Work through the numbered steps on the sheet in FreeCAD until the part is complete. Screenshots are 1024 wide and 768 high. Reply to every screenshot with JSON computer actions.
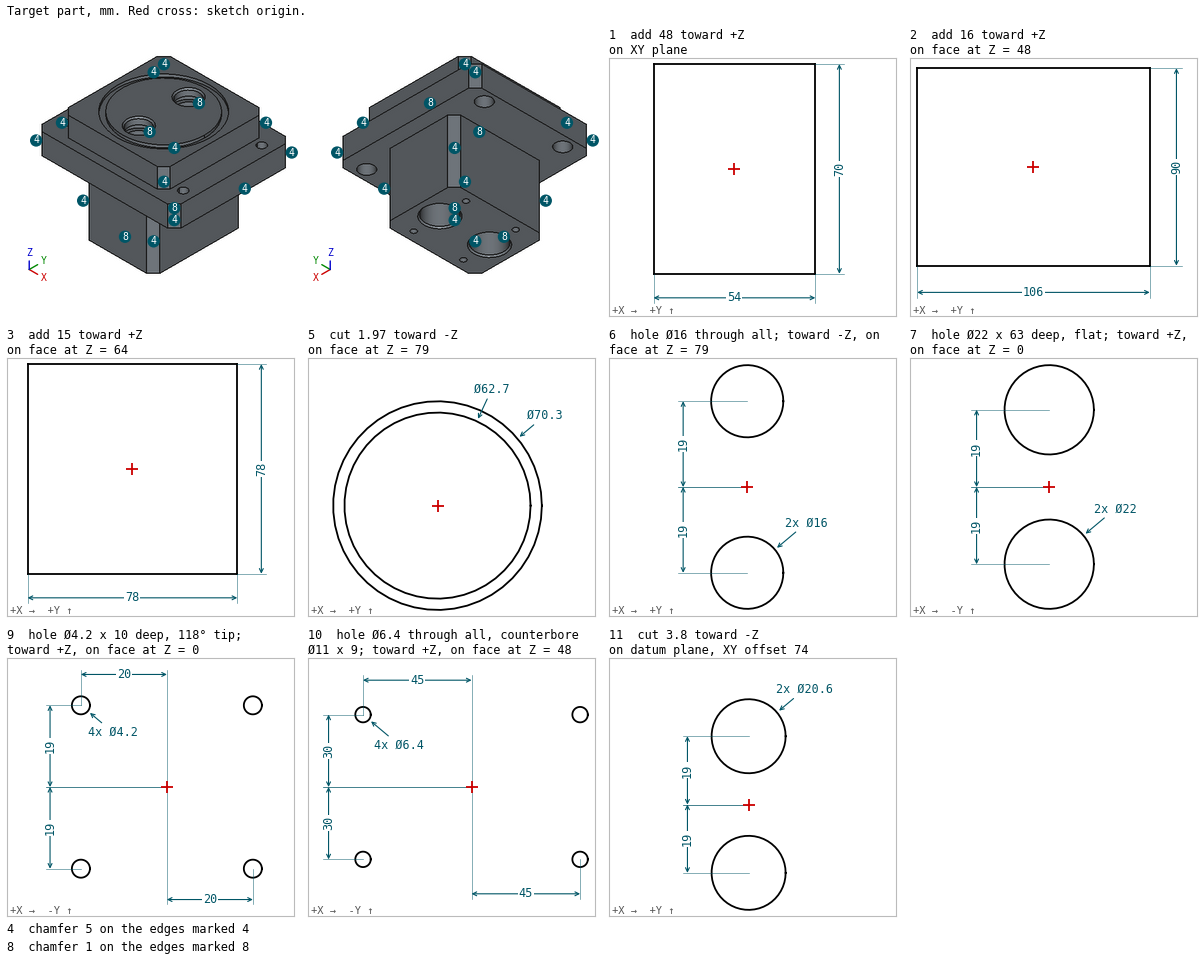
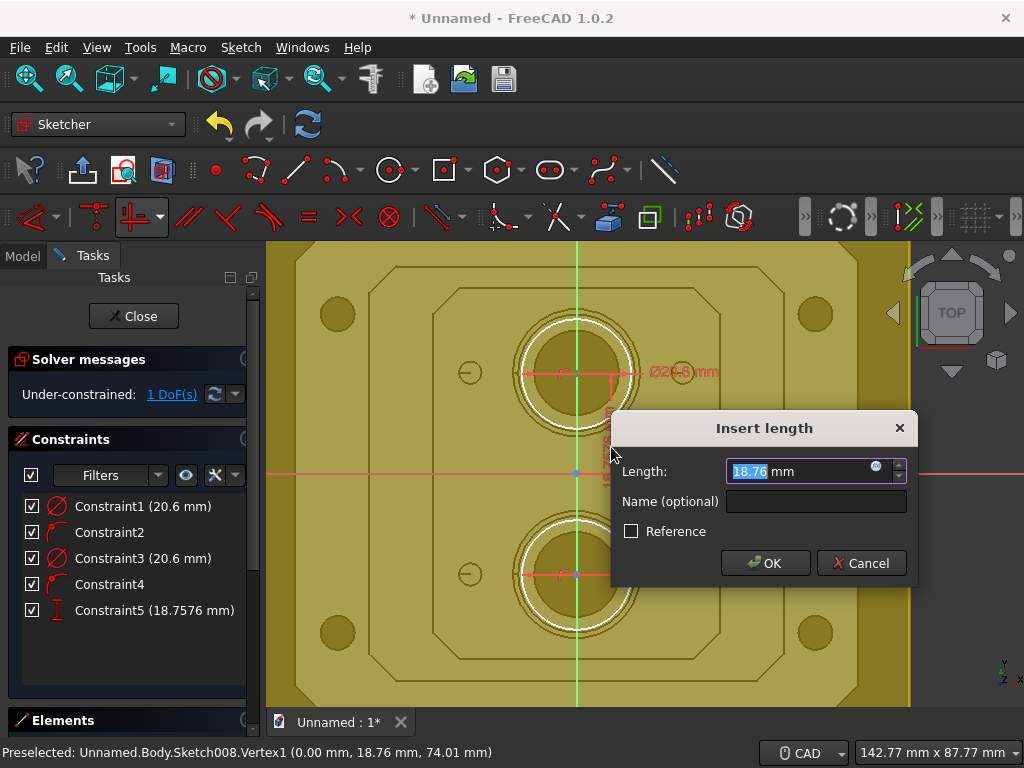
{"action": "type", "text": "19"}
{"action": "key", "text": "Return"}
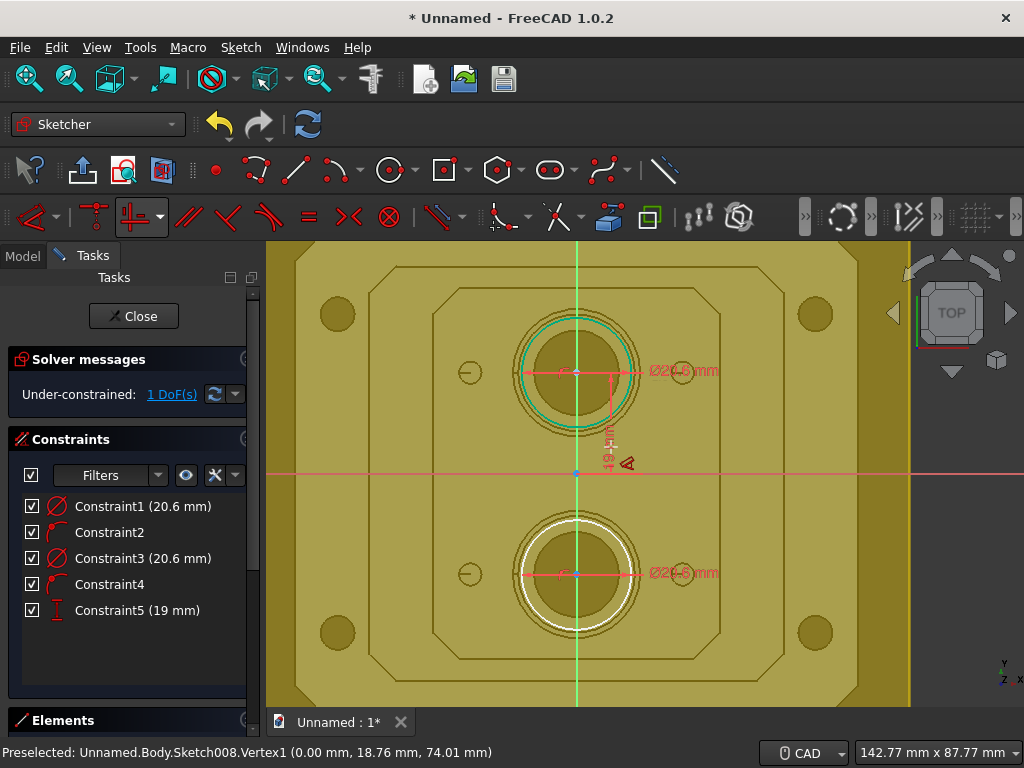
{"action": "left_click", "coordinate": [577, 575]}
{"action": "left_click", "coordinate": [611, 501]}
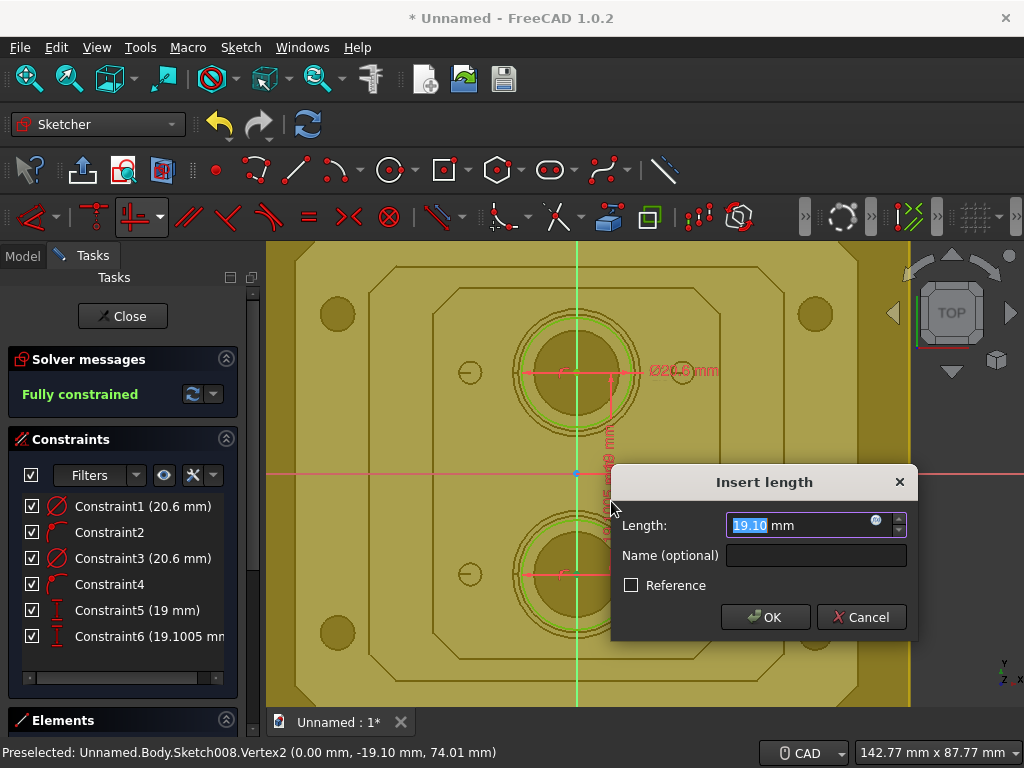
{"action": "type", "text": "19"}
{"action": "key", "text": "Return"}
{"action": "key", "text": "Escape"}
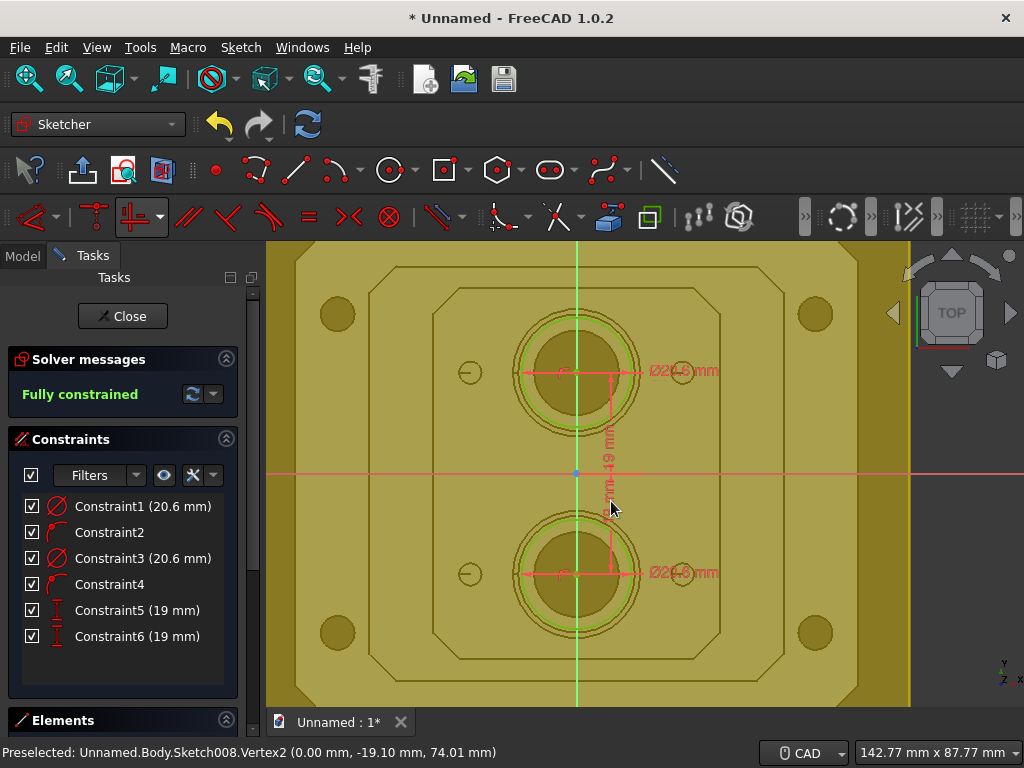
{"action": "left_click", "coordinate": [123, 316]}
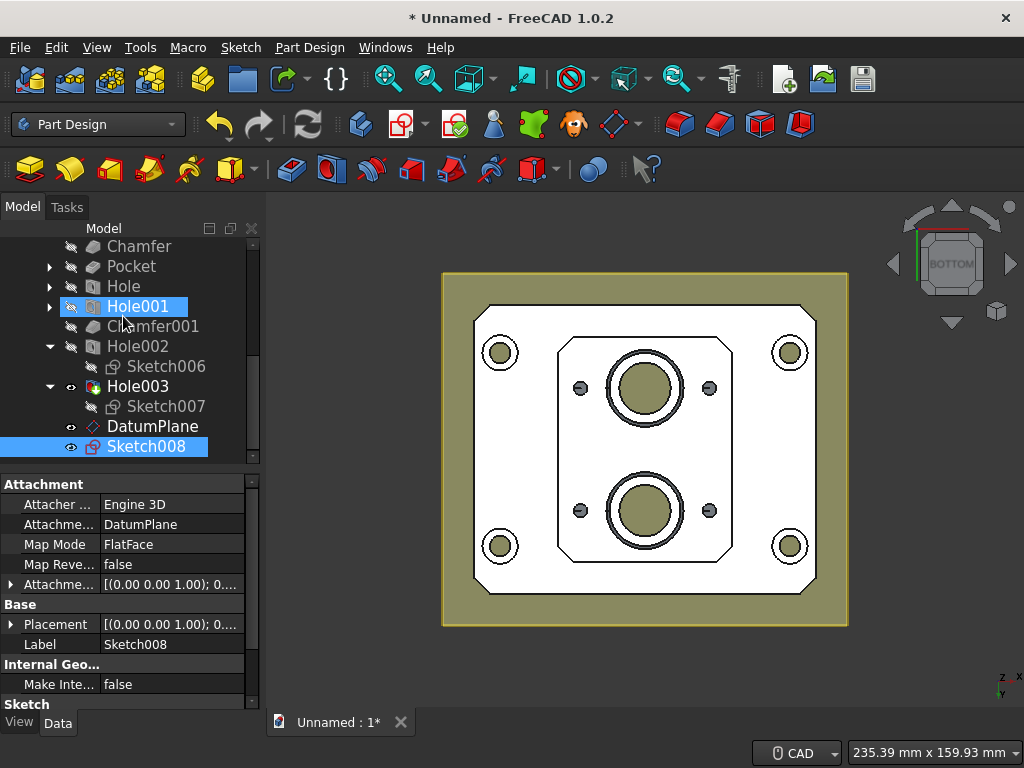
{"action": "left_click", "coordinate": [292, 170]}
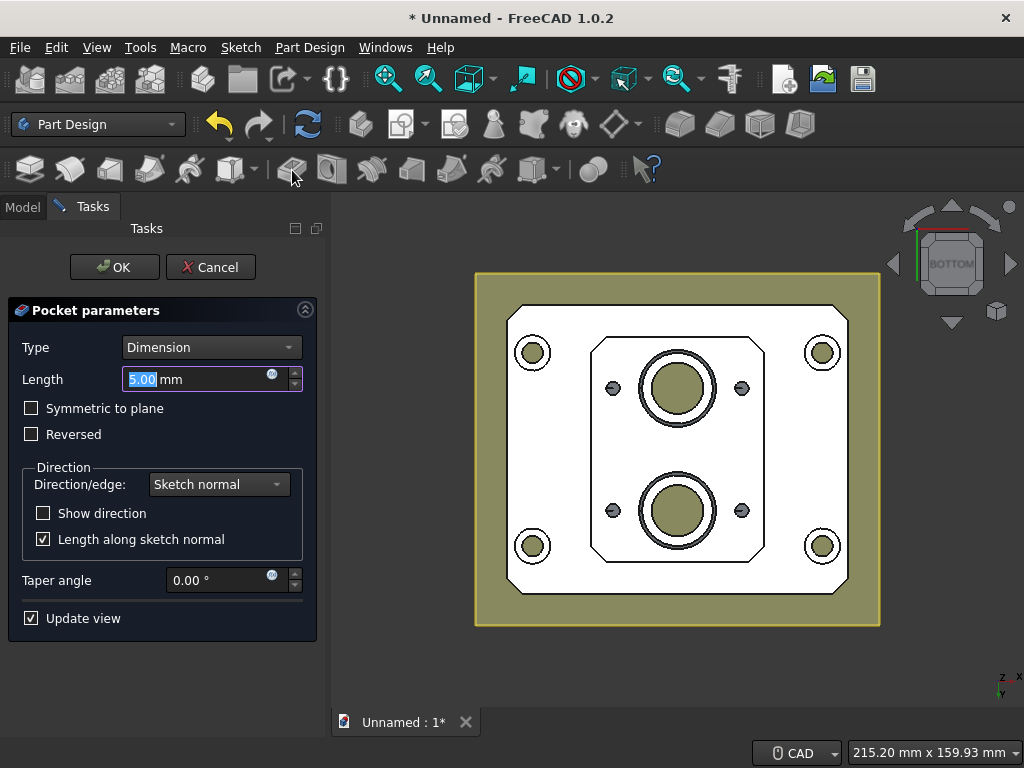
{"action": "type", "text": "3.8"}
{"action": "key", "text": "Tab"}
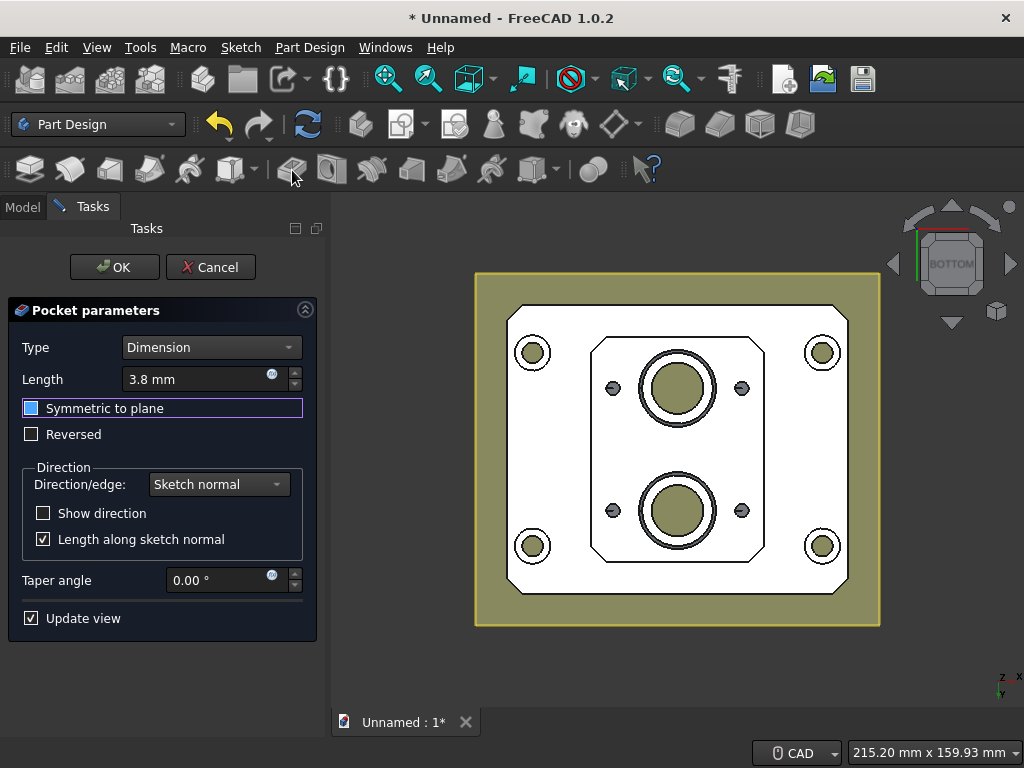
{"action": "left_click", "coordinate": [115, 267]}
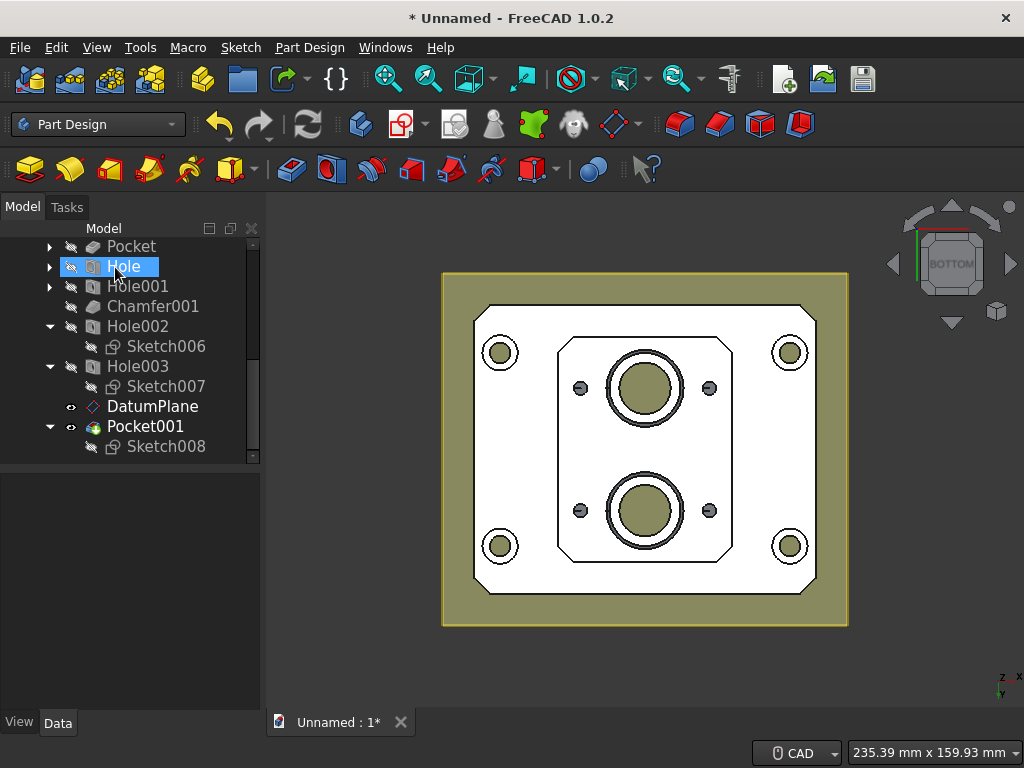
{"action": "left_click", "coordinate": [116, 407]}
{"action": "key", "text": "space"}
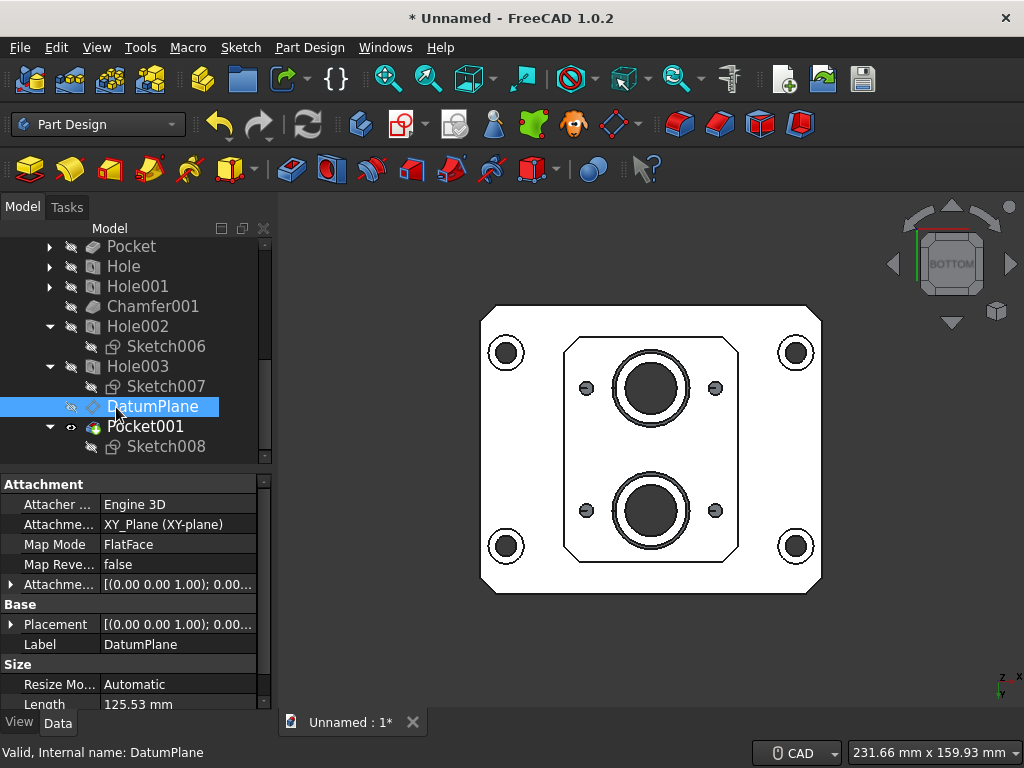
{"action": "key", "text": "0"}